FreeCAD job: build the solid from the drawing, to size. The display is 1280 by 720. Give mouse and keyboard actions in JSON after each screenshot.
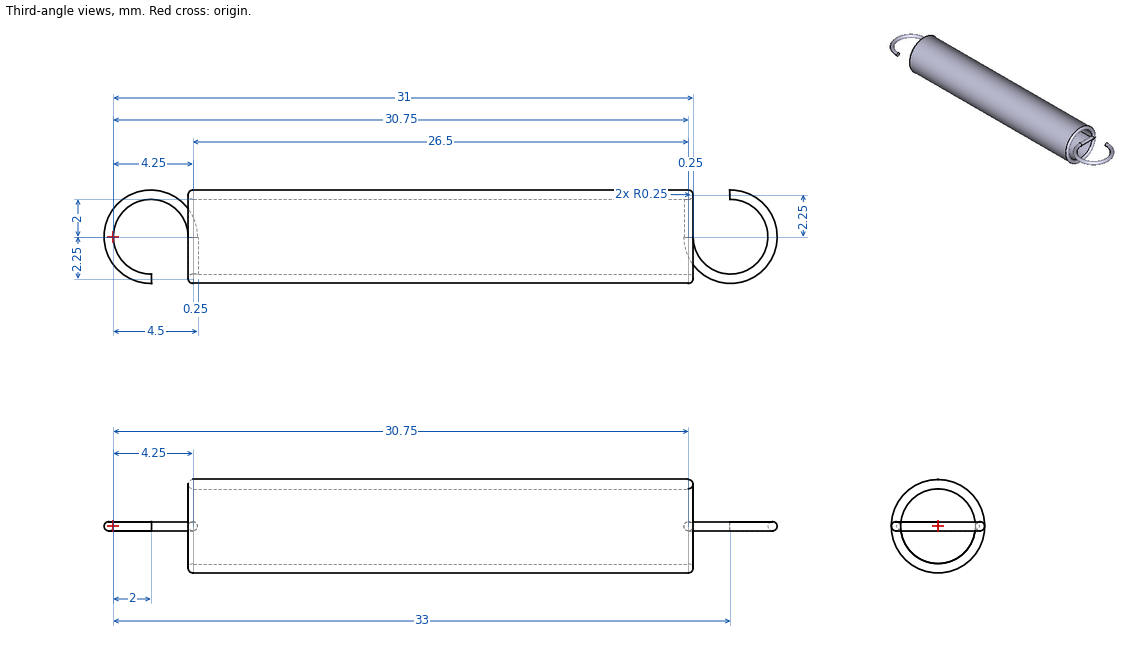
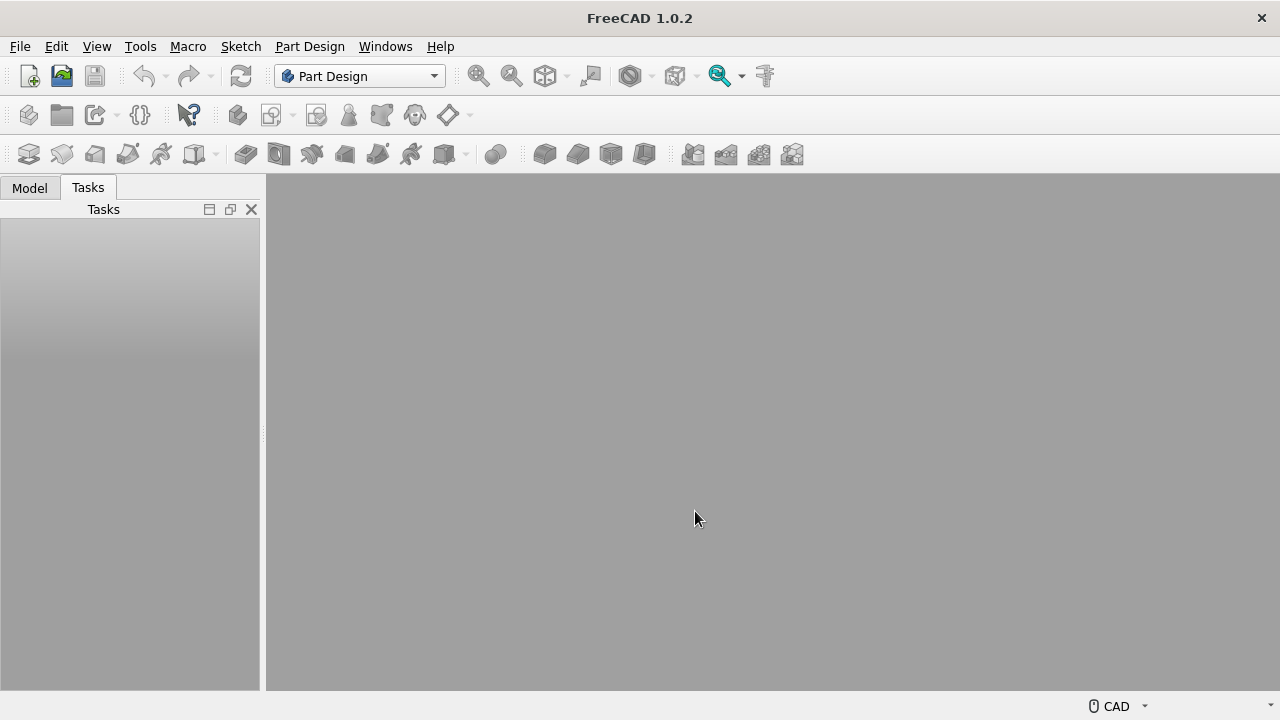
{"action": "left_click", "coordinate": [29, 76]}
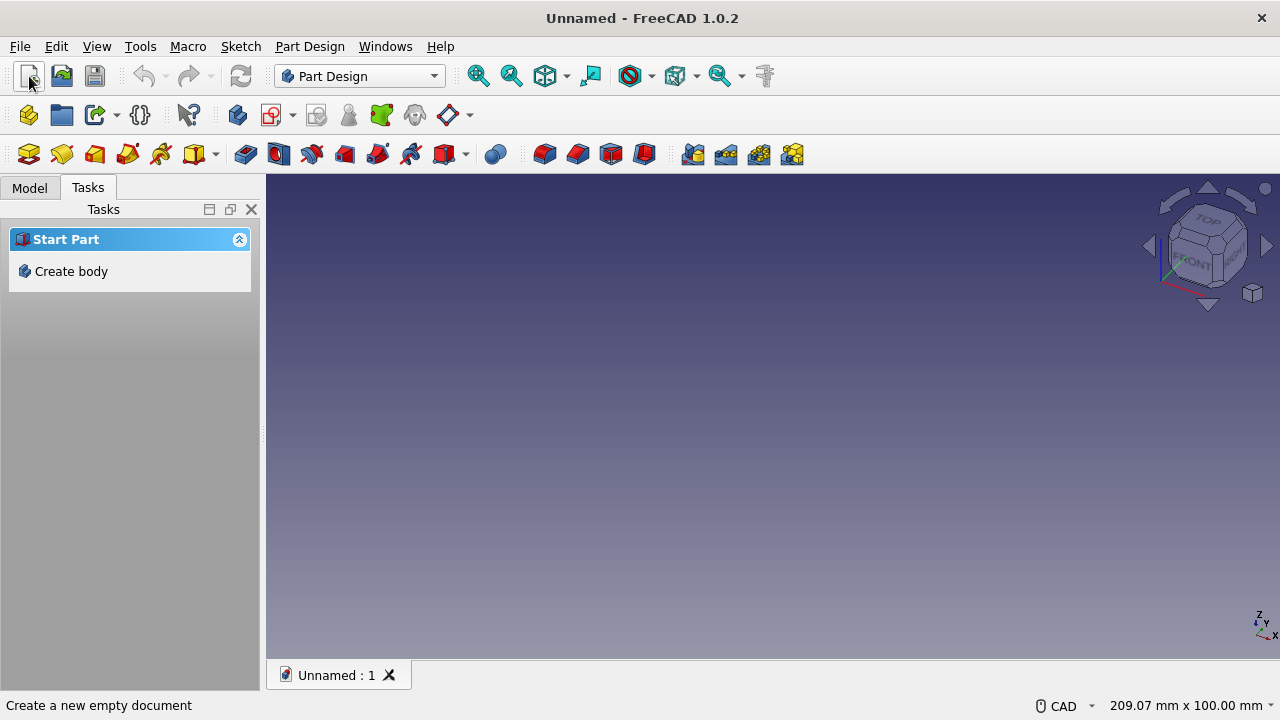
{"action": "left_click", "coordinate": [270, 116]}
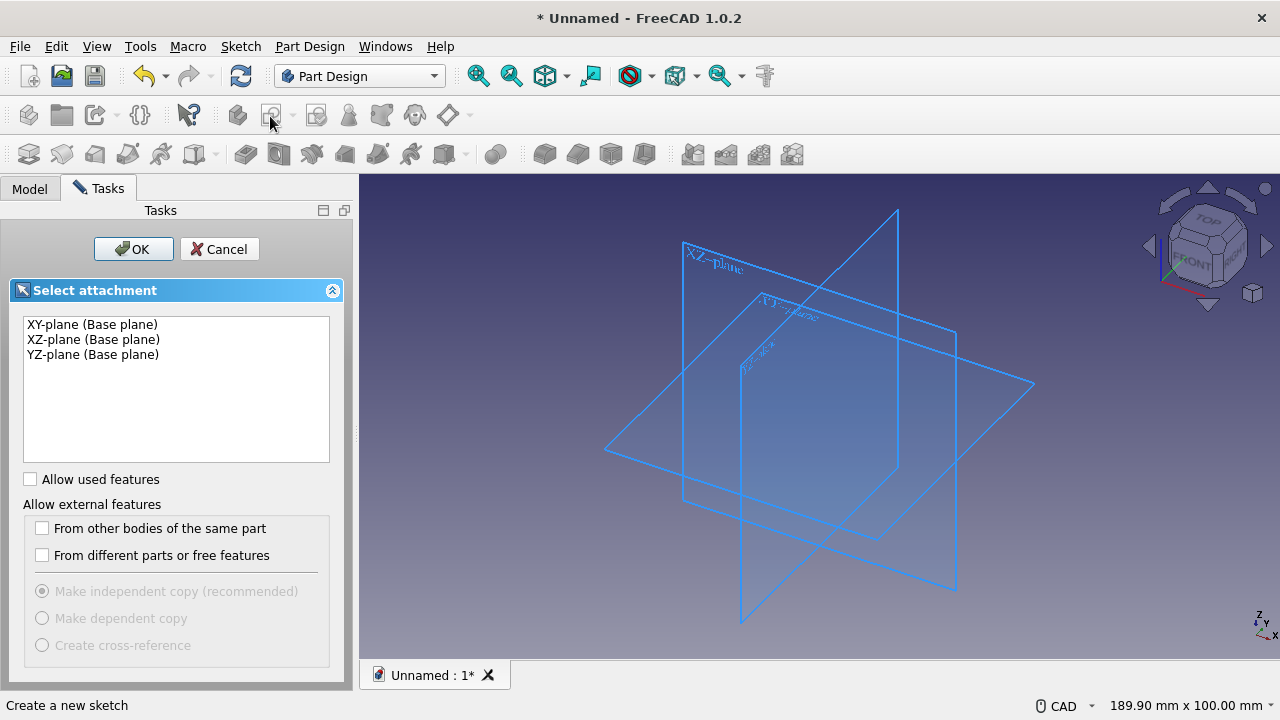
{"action": "left_click", "coordinate": [84, 324]}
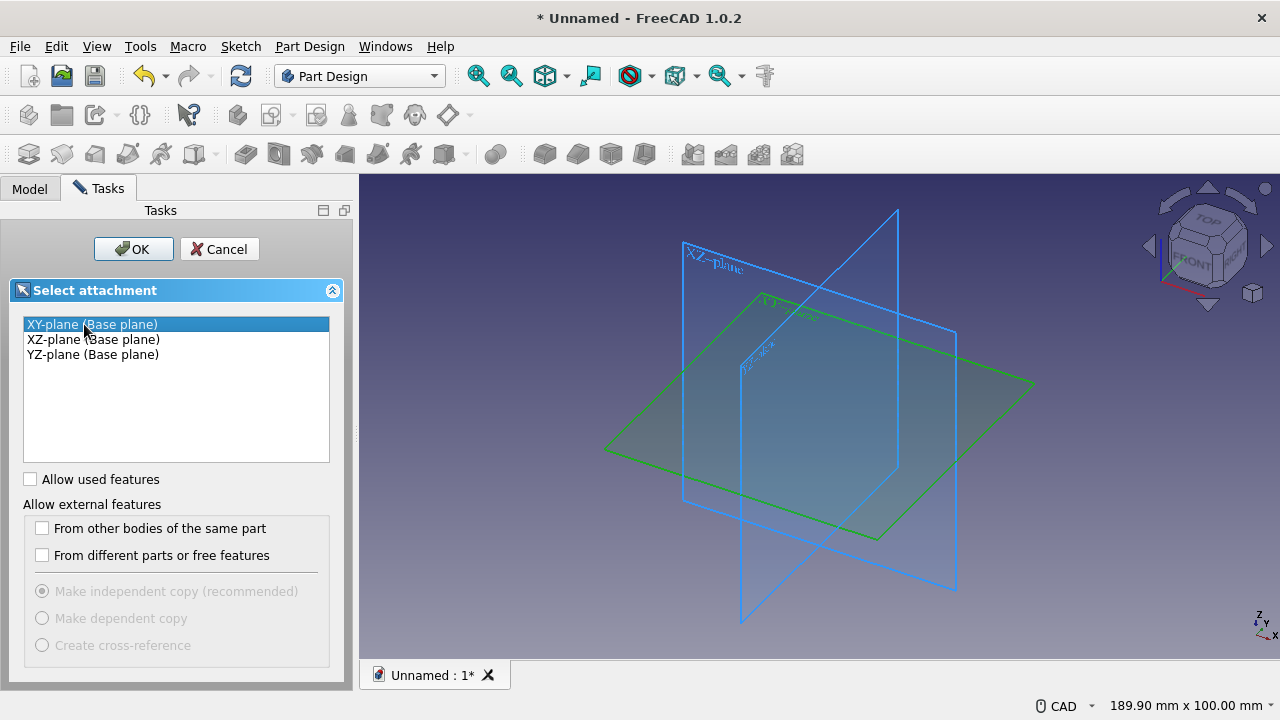
{"action": "left_click", "coordinate": [134, 249]}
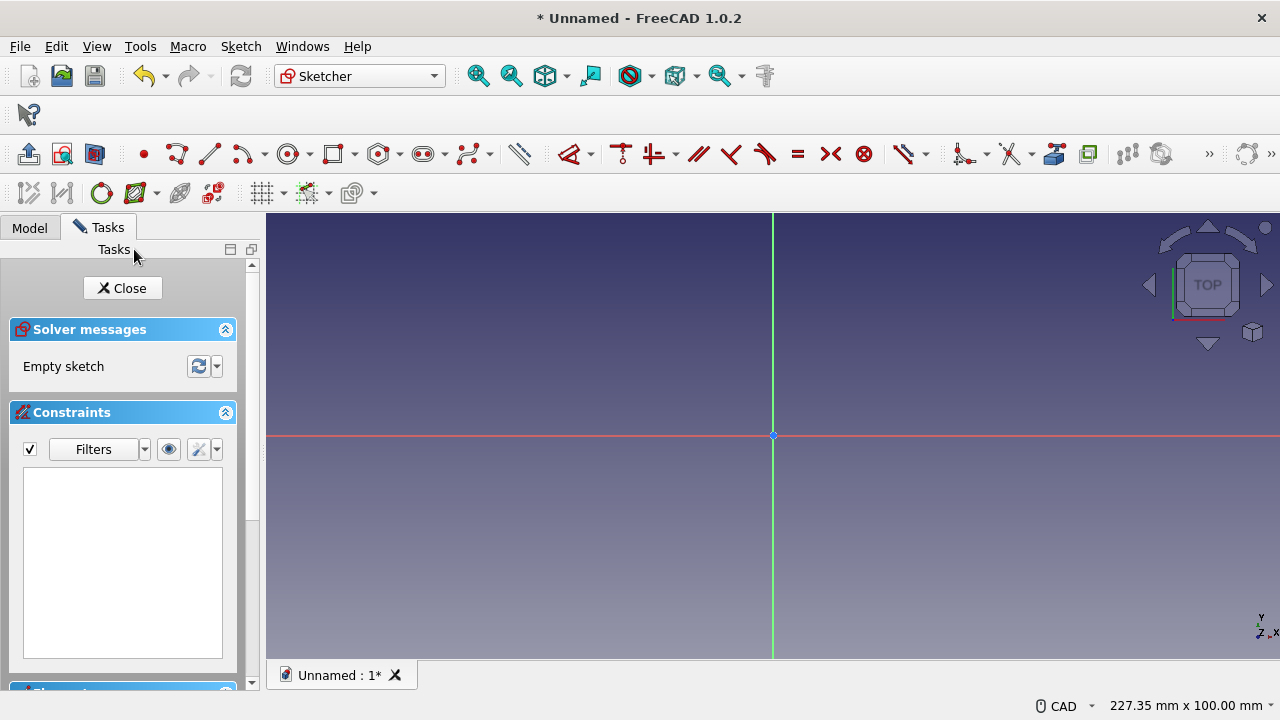
{"action": "scroll", "coordinate": [887, 429], "scroll_direction": "up", "scroll_amount": 7}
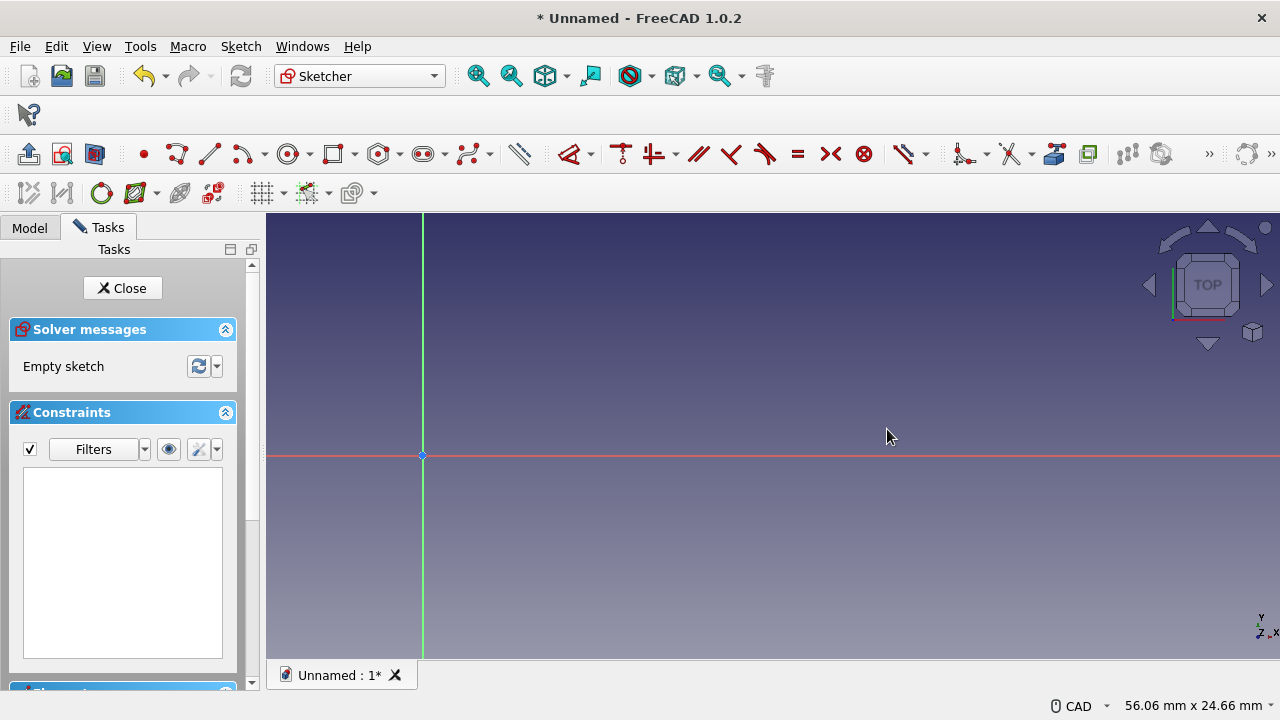
{"action": "key", "text": "g s"}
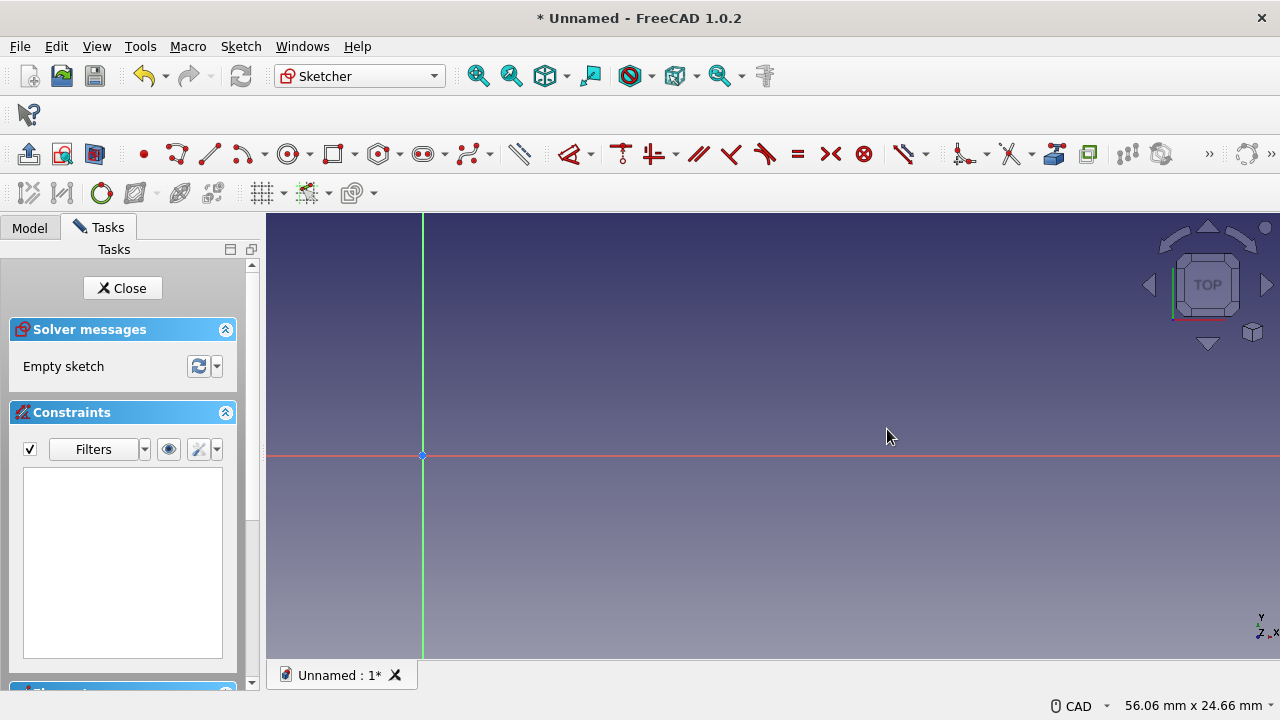
{"action": "scroll", "coordinate": [500, 415], "scroll_direction": "up", "scroll_amount": 9}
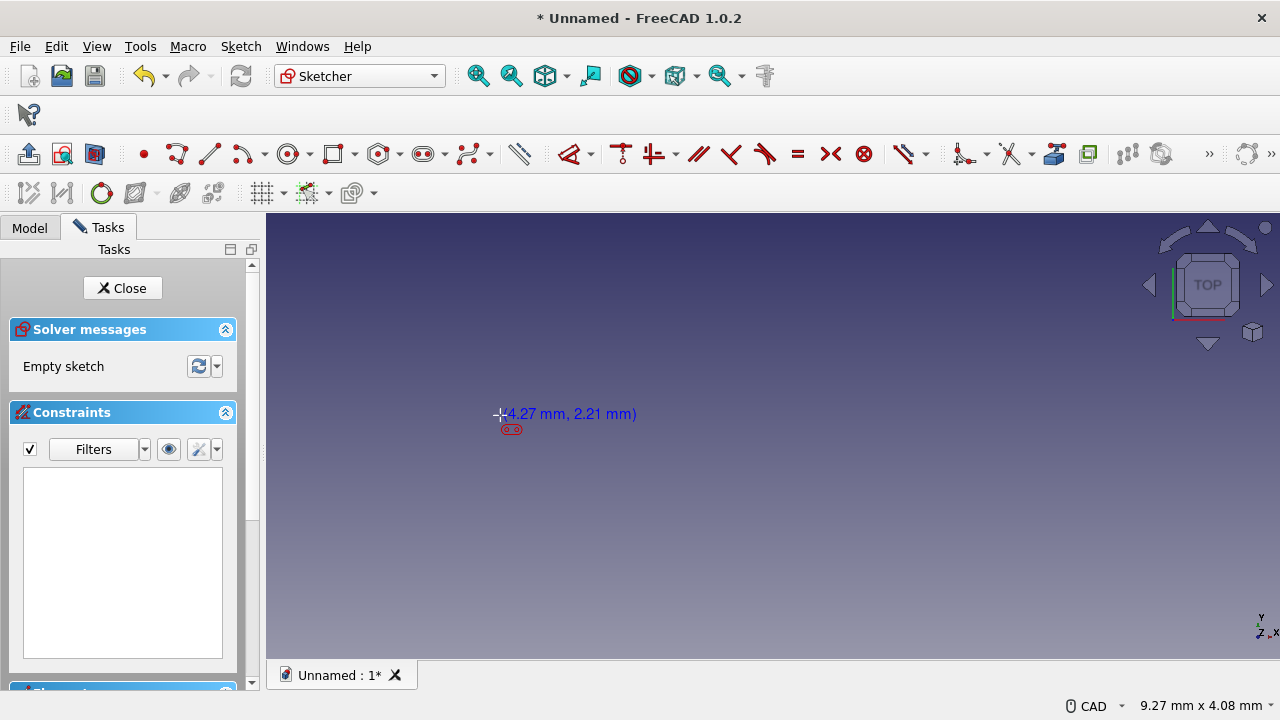
{"action": "scroll", "coordinate": [502, 419], "scroll_direction": "down", "scroll_amount": 9}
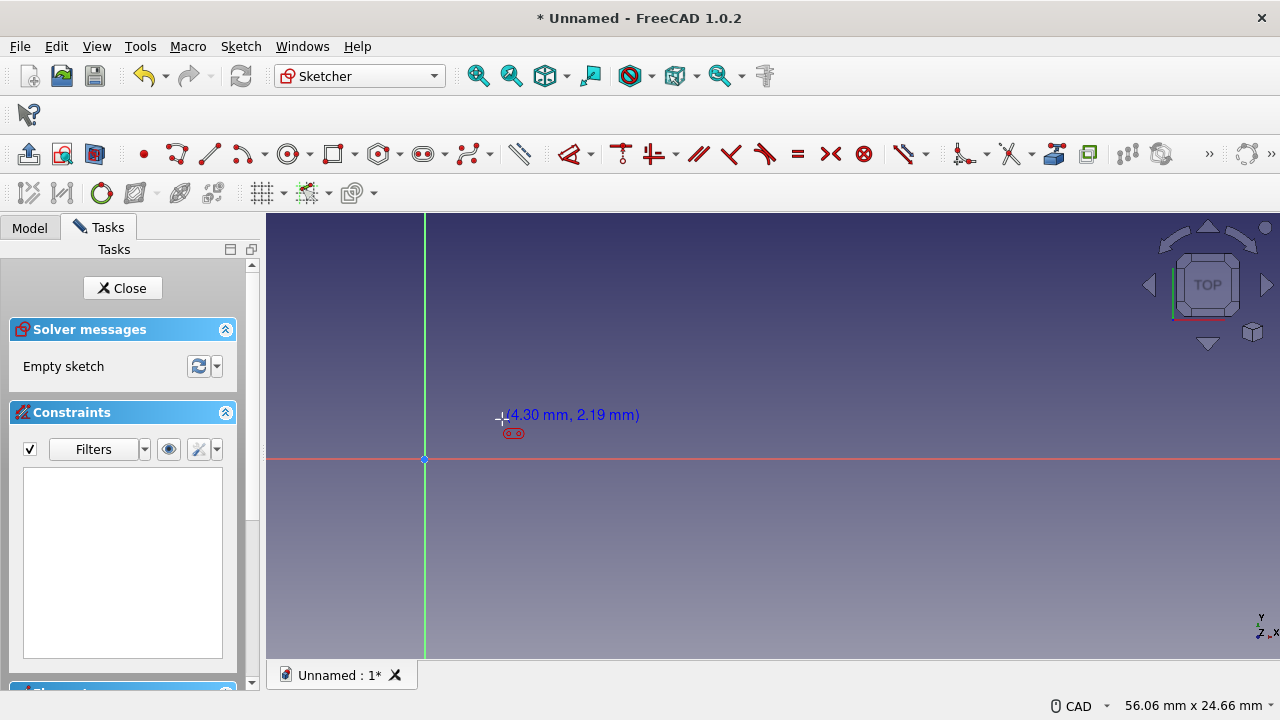
{"action": "left_click", "coordinate": [501, 419]}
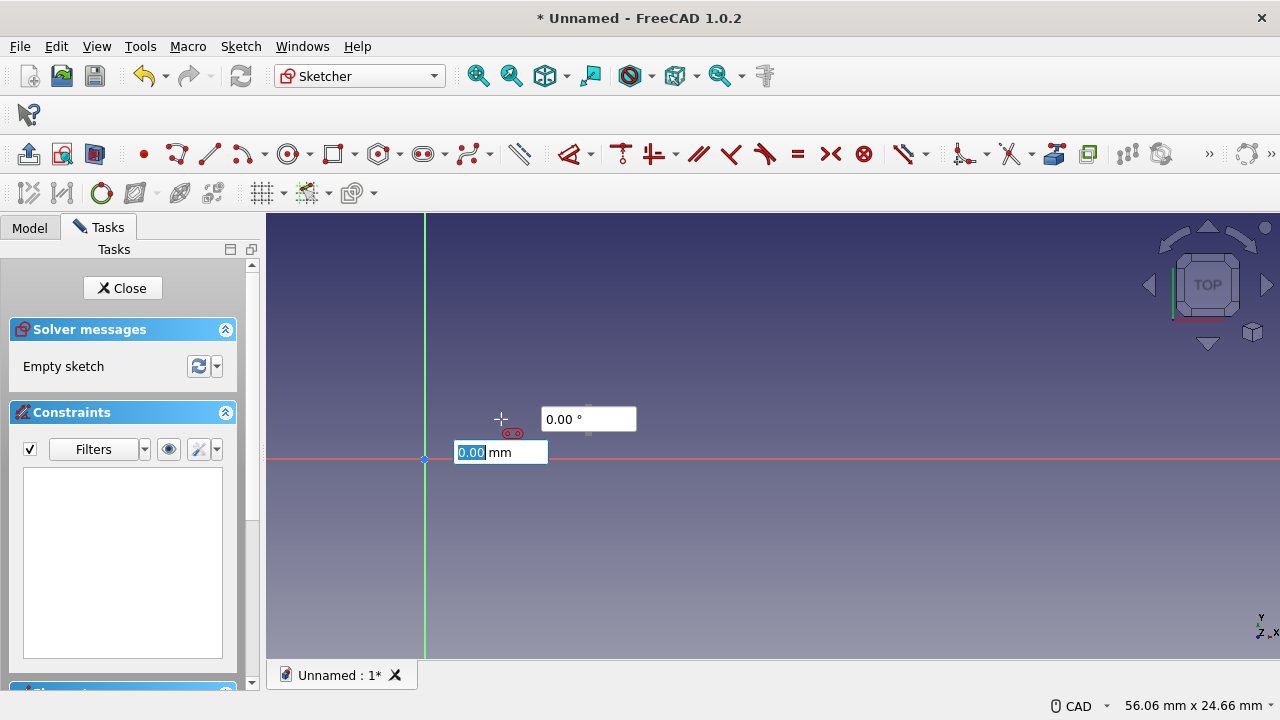
{"action": "left_click", "coordinate": [981, 419]}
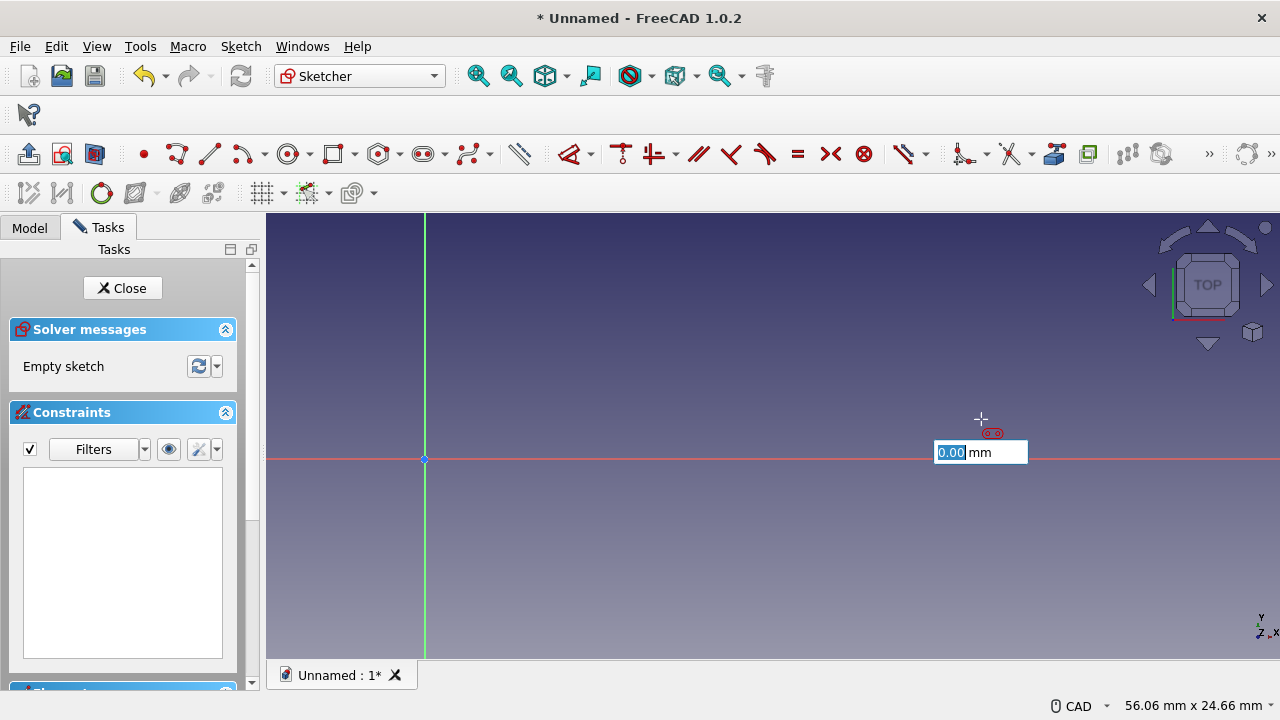
{"action": "scroll", "coordinate": [741, 423], "scroll_direction": "up", "scroll_amount": 7}